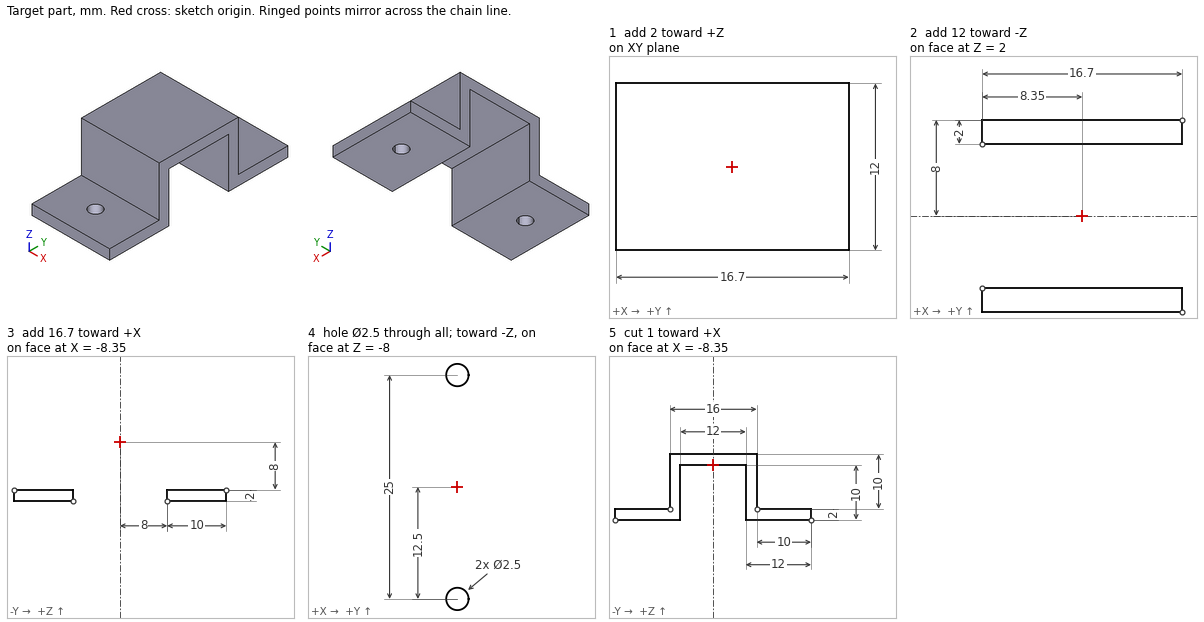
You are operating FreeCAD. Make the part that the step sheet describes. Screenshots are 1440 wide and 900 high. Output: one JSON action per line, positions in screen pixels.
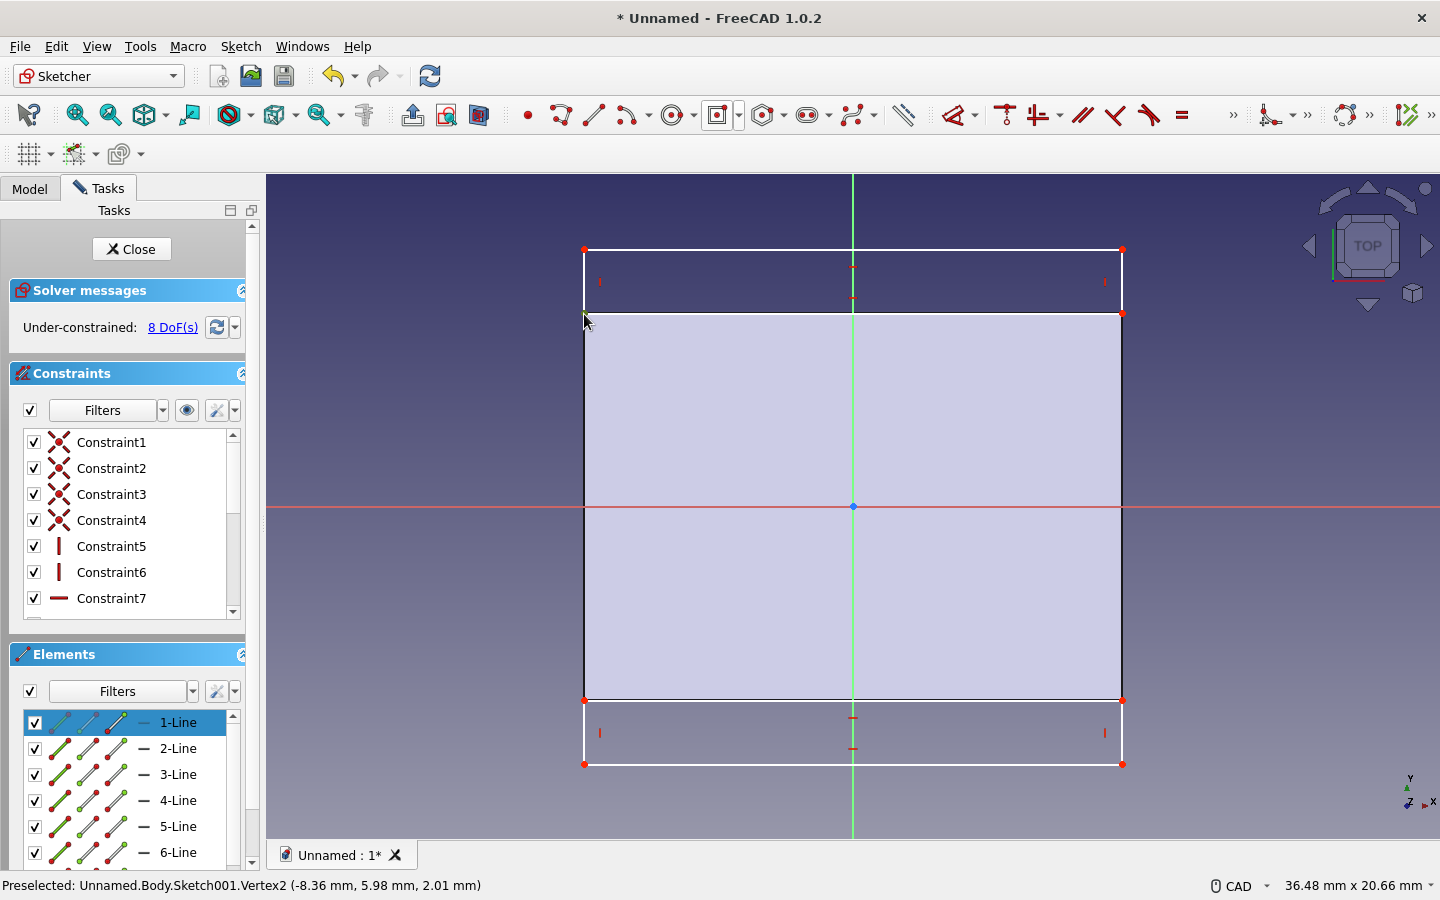
{"action": "left_click", "coordinate": [584, 701]}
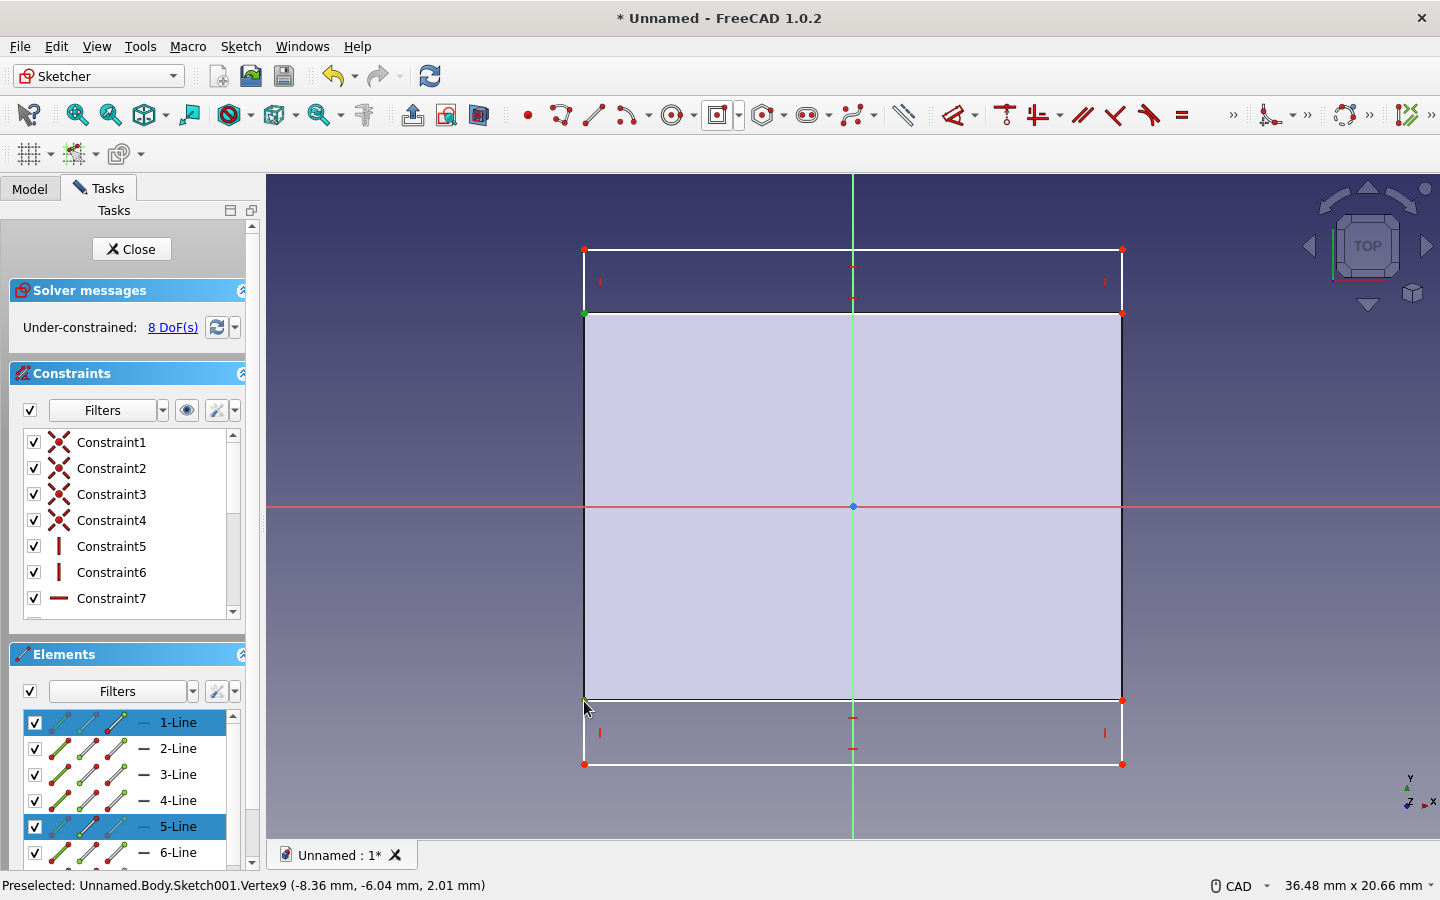
{"action": "left_click", "coordinate": [364, 506]}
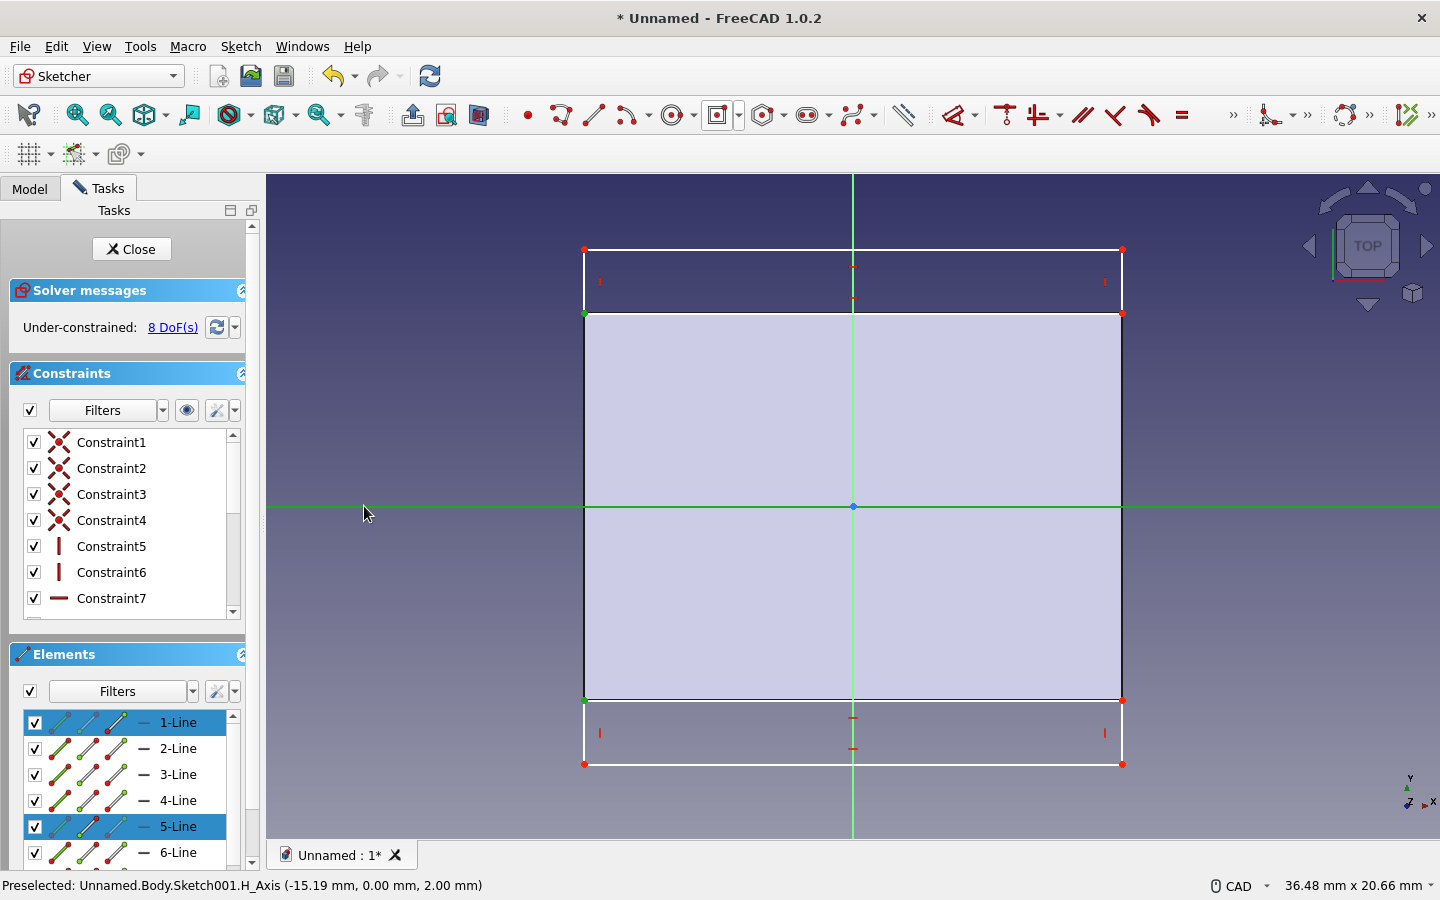
{"action": "key", "text": "s"}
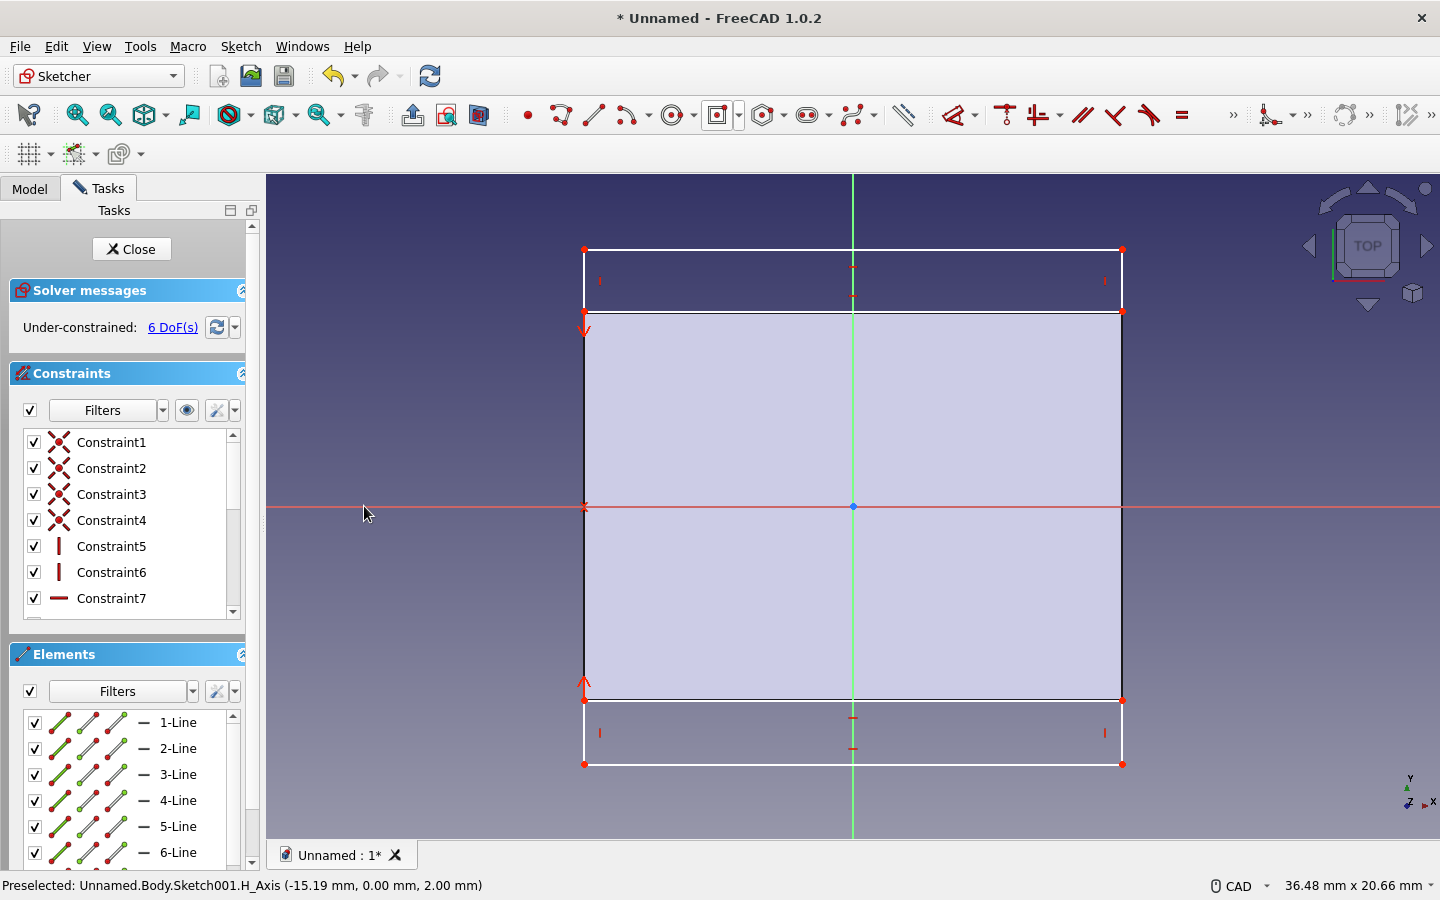
{"action": "left_click", "coordinate": [1122, 250]}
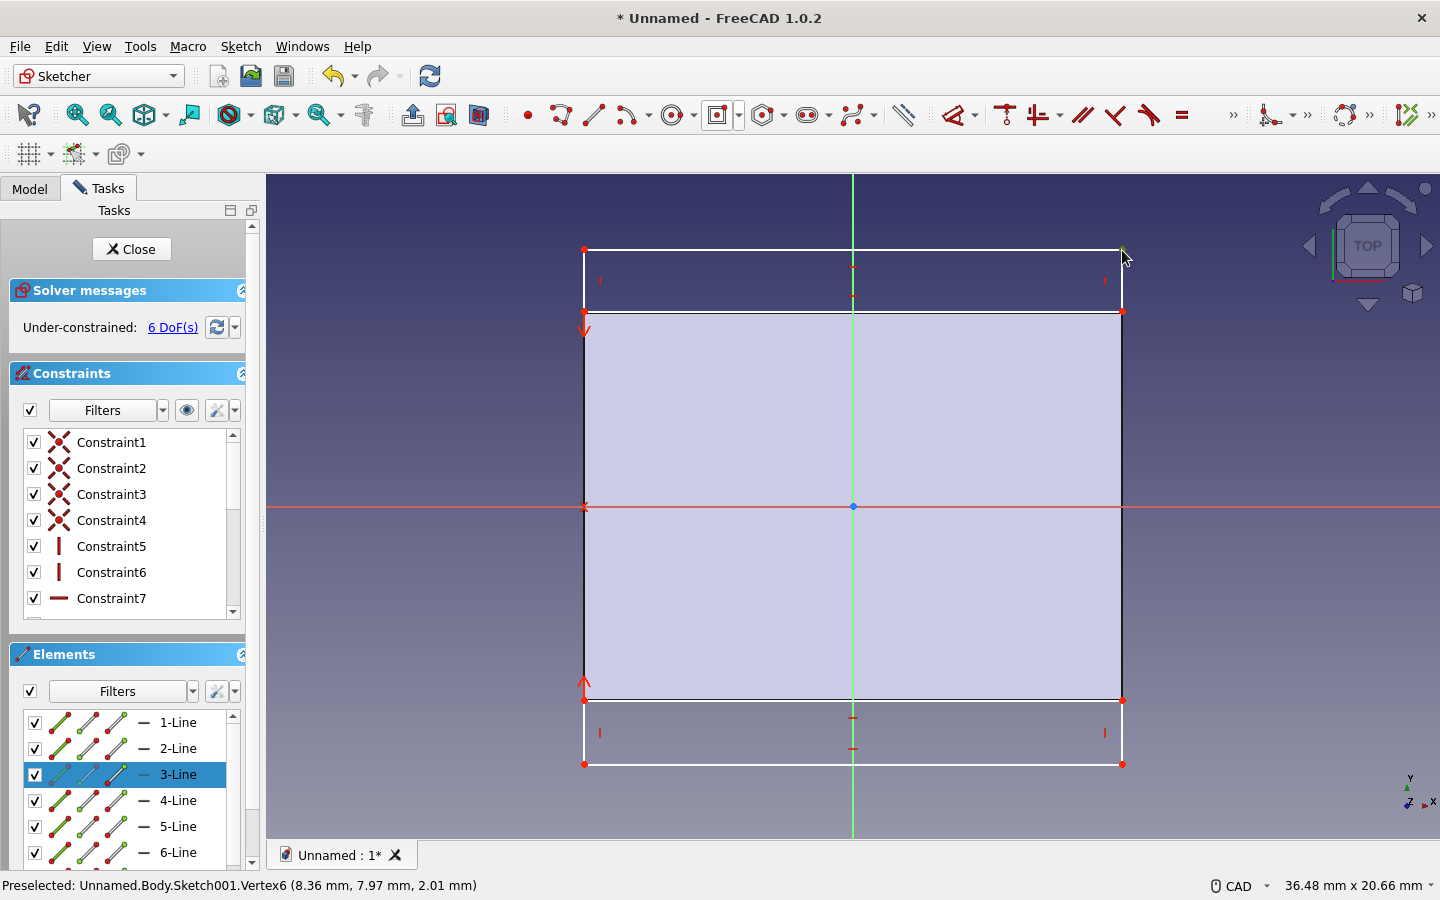
{"action": "left_click", "coordinate": [1122, 765]}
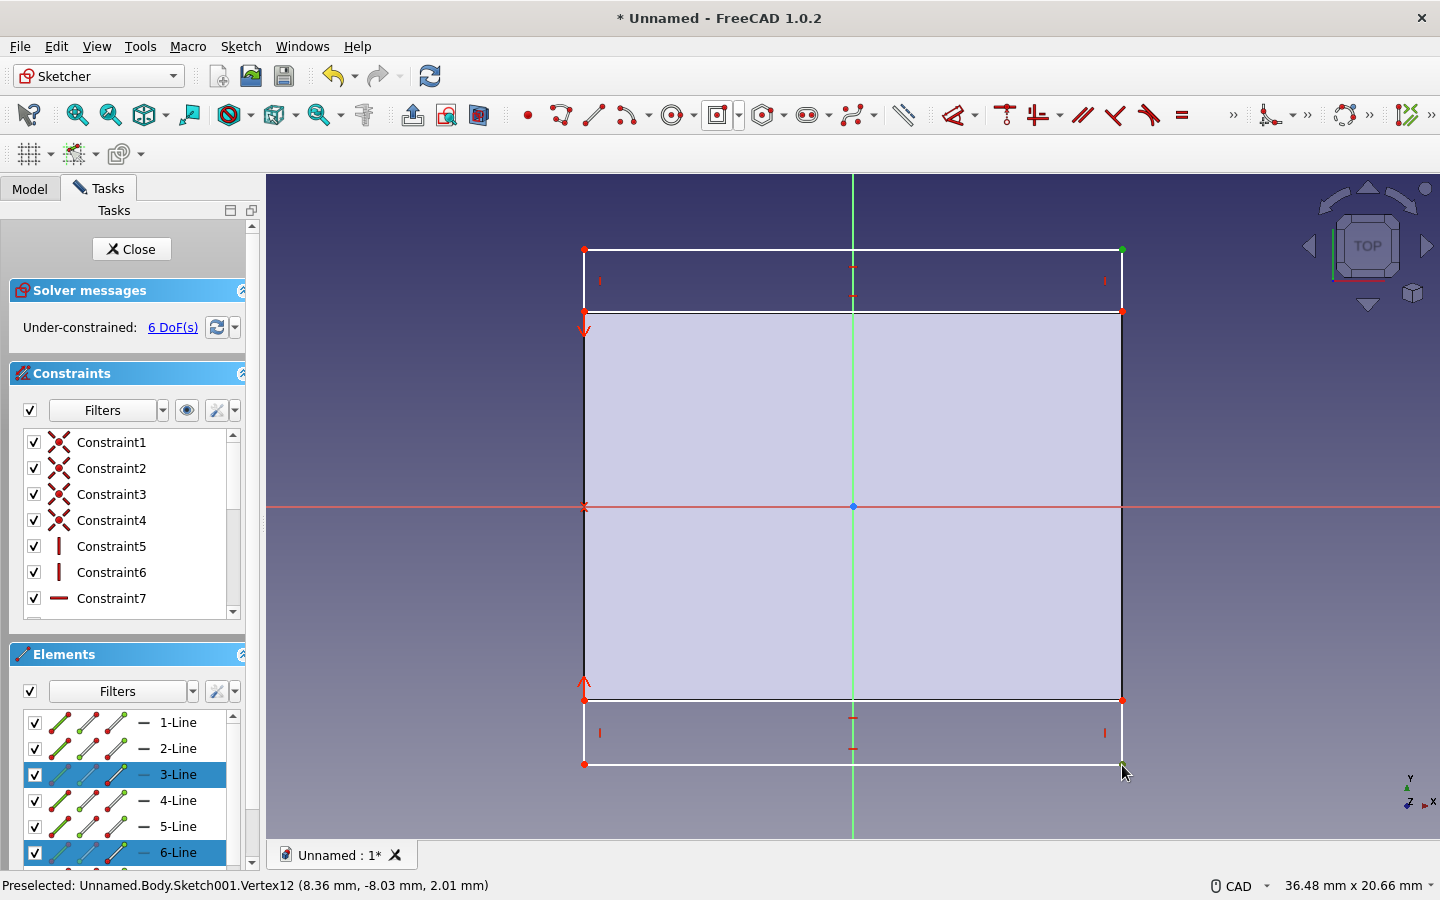
{"action": "left_click", "coordinate": [364, 506]}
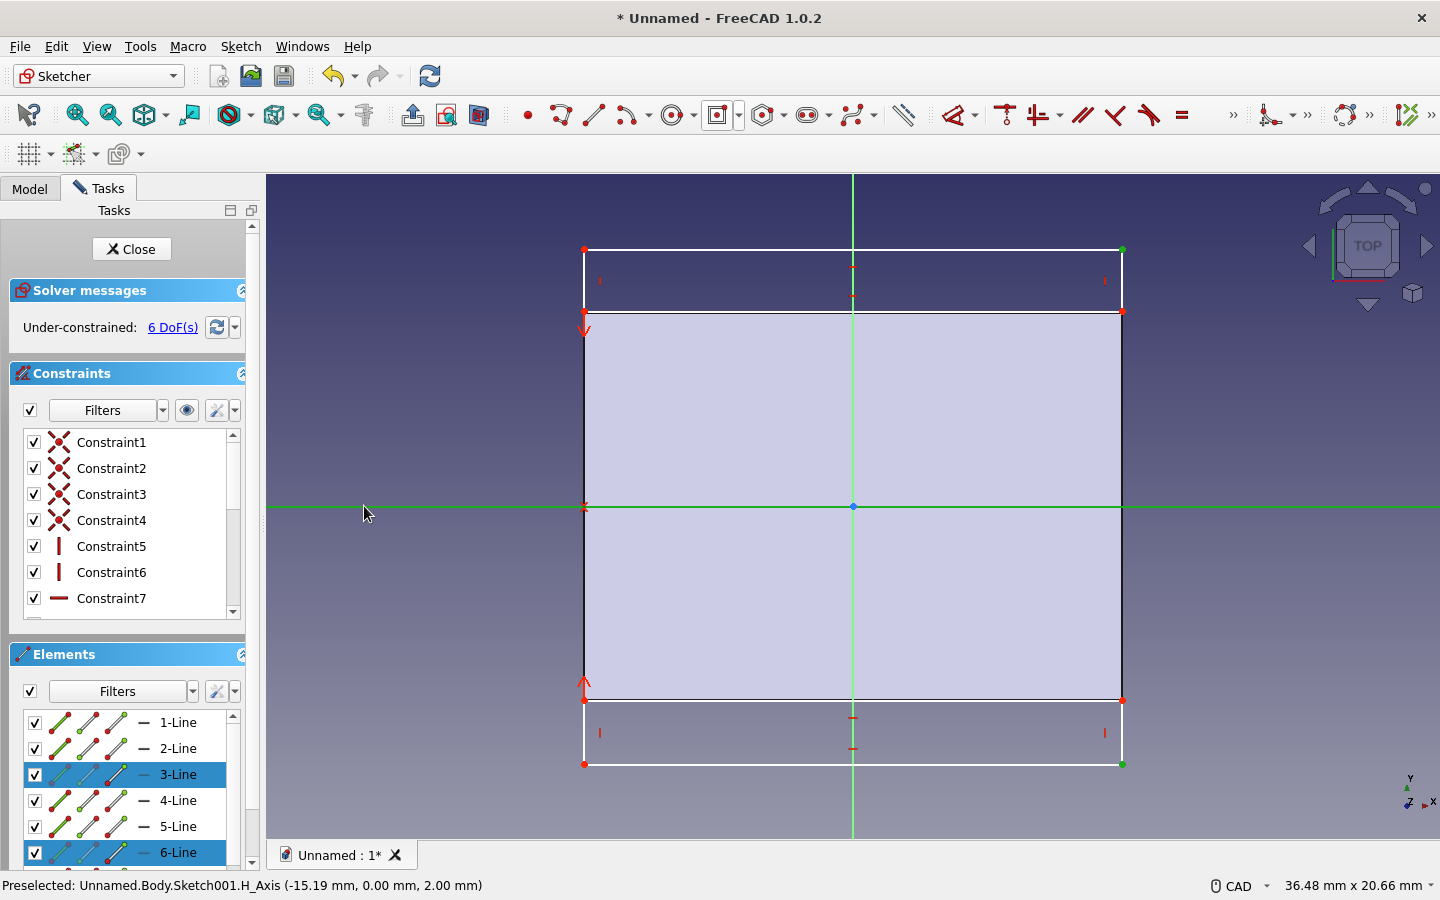
{"action": "key", "text": "s"}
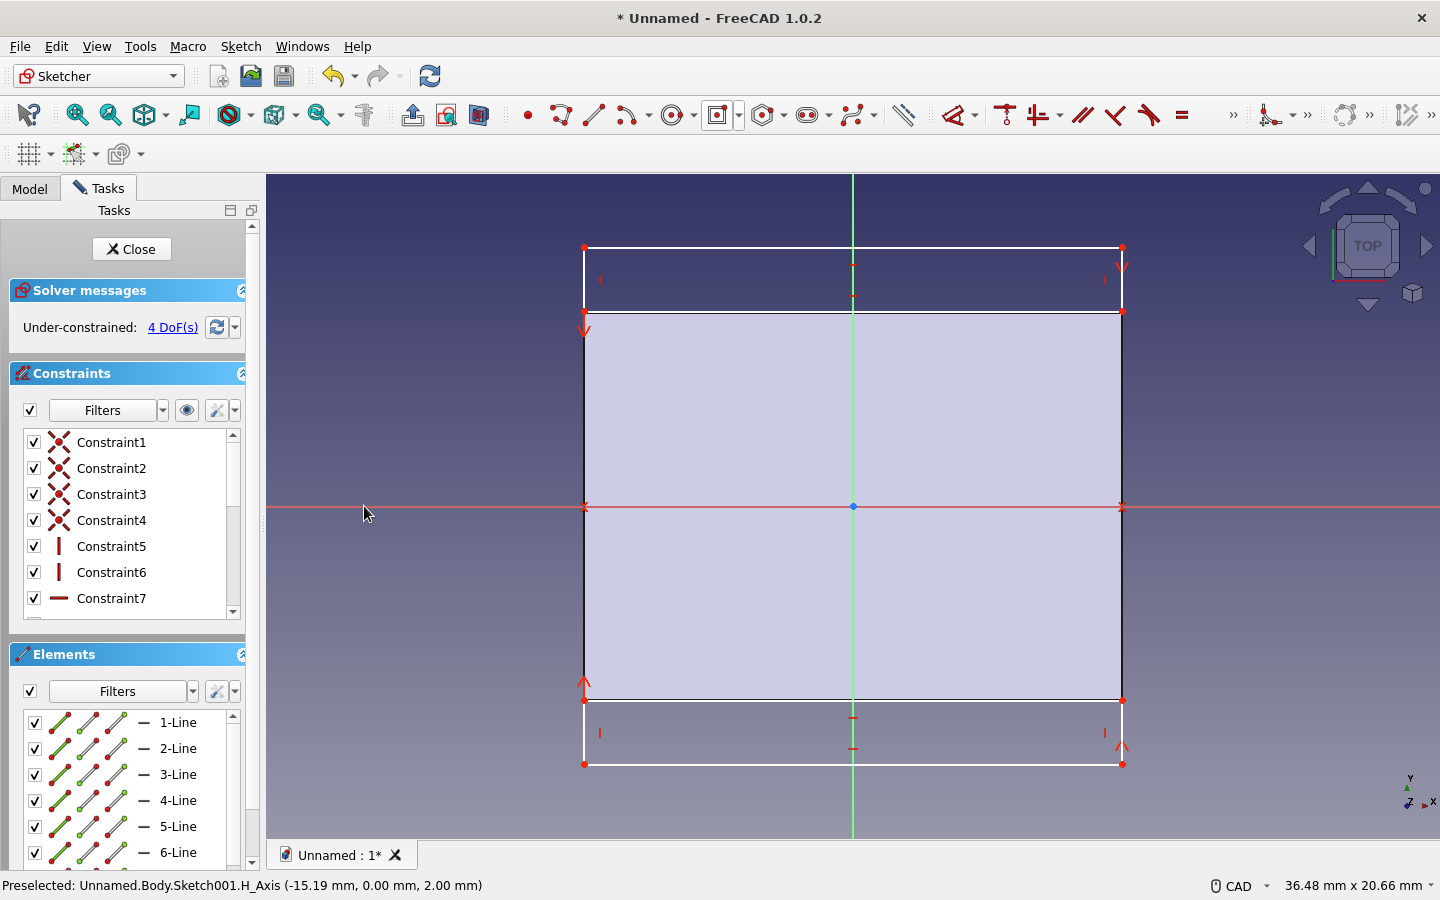
{"action": "left_click", "coordinate": [952, 116]}